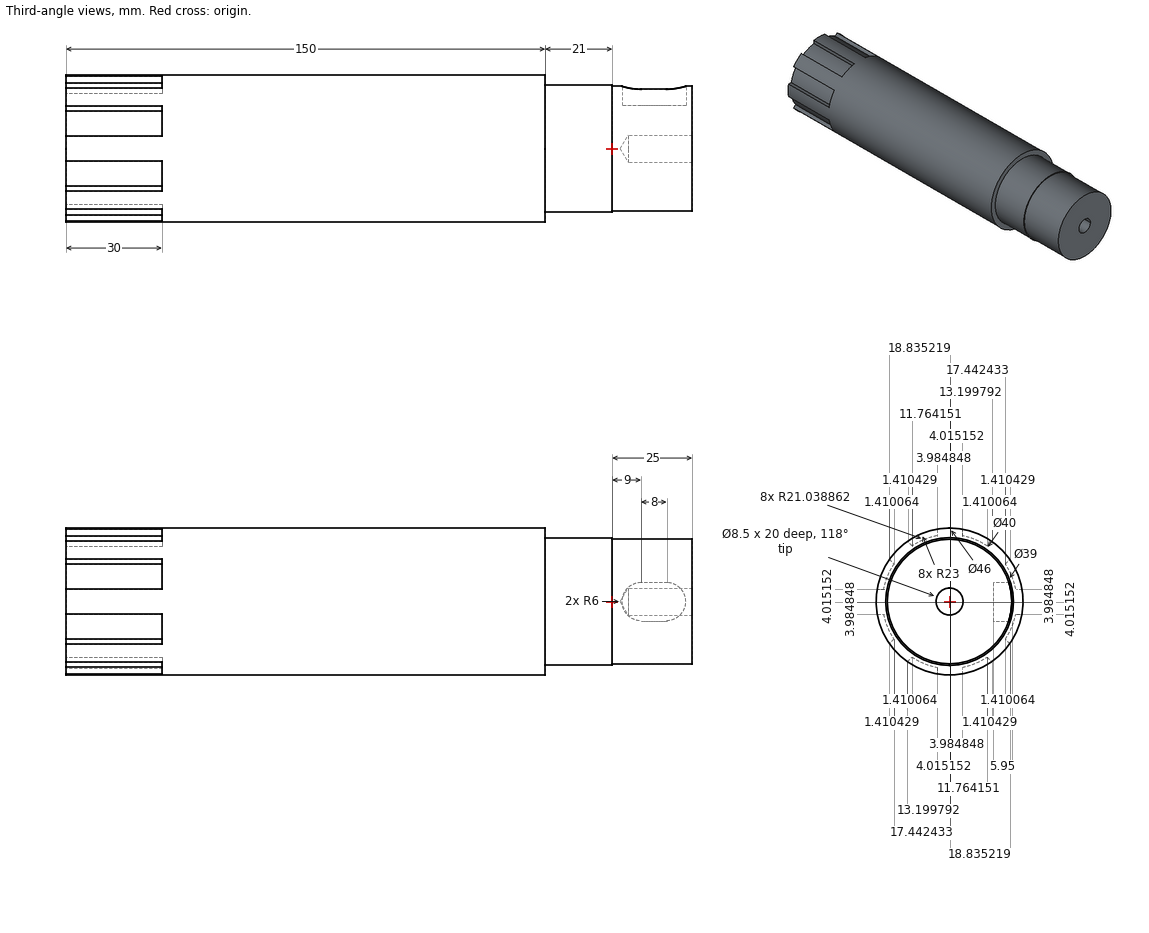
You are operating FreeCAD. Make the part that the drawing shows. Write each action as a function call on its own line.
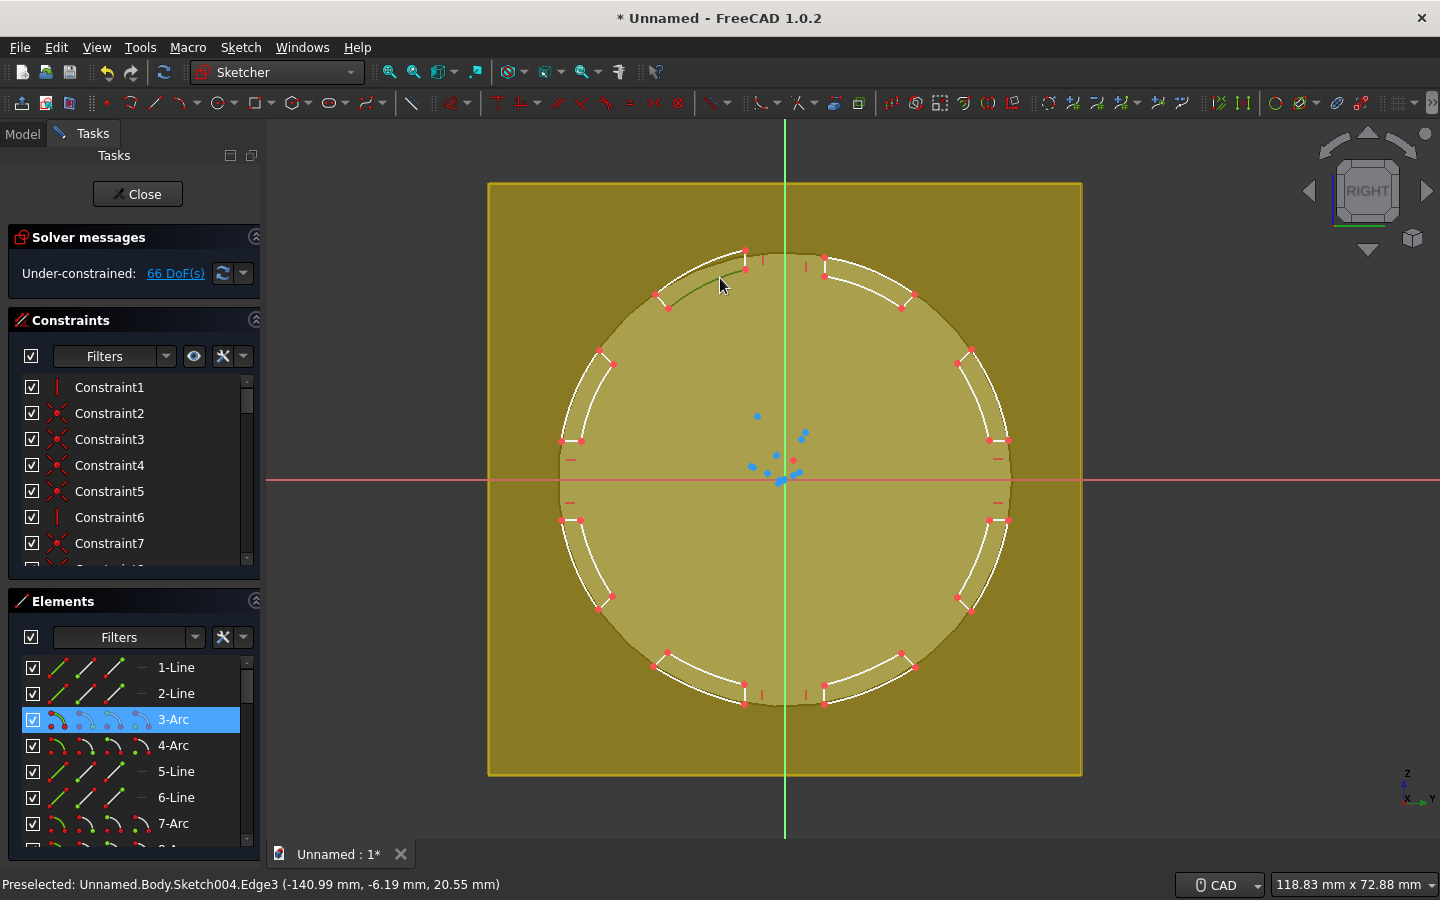
click(680, 681)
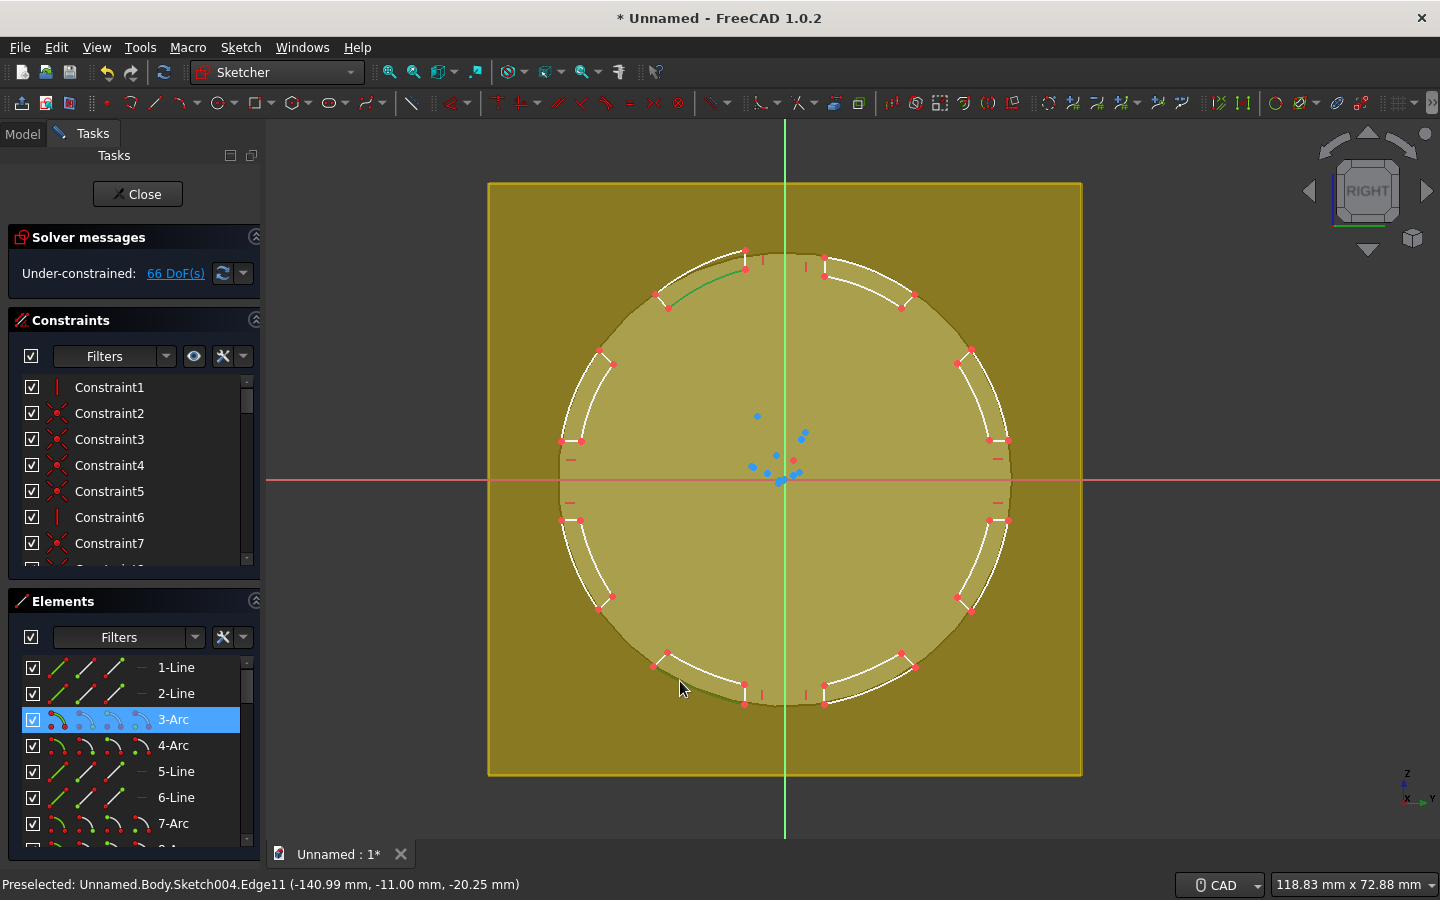
click(498, 104)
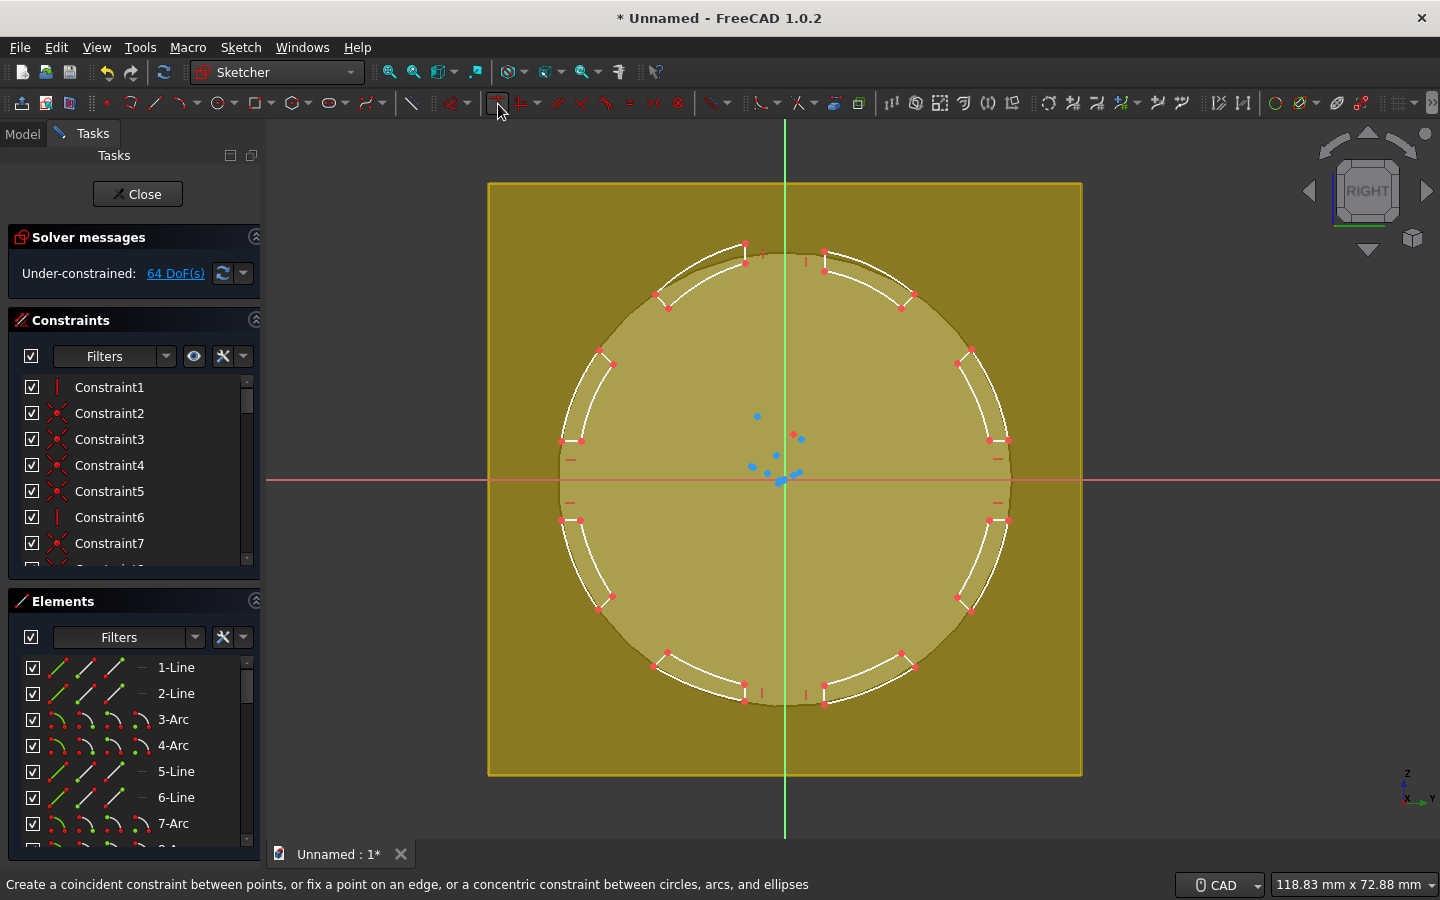
click(720, 273)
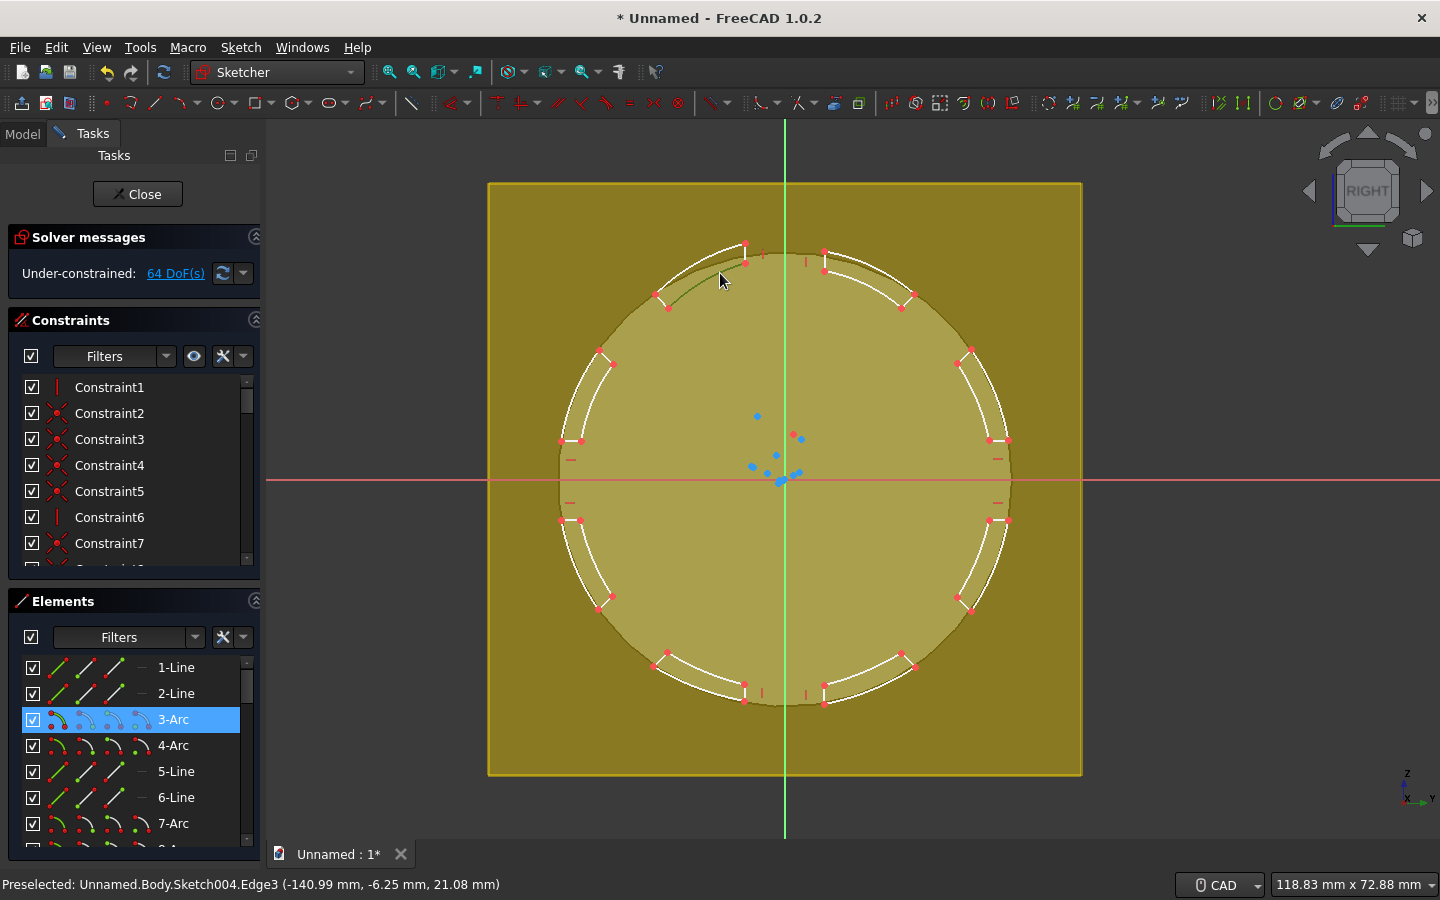
click(690, 665)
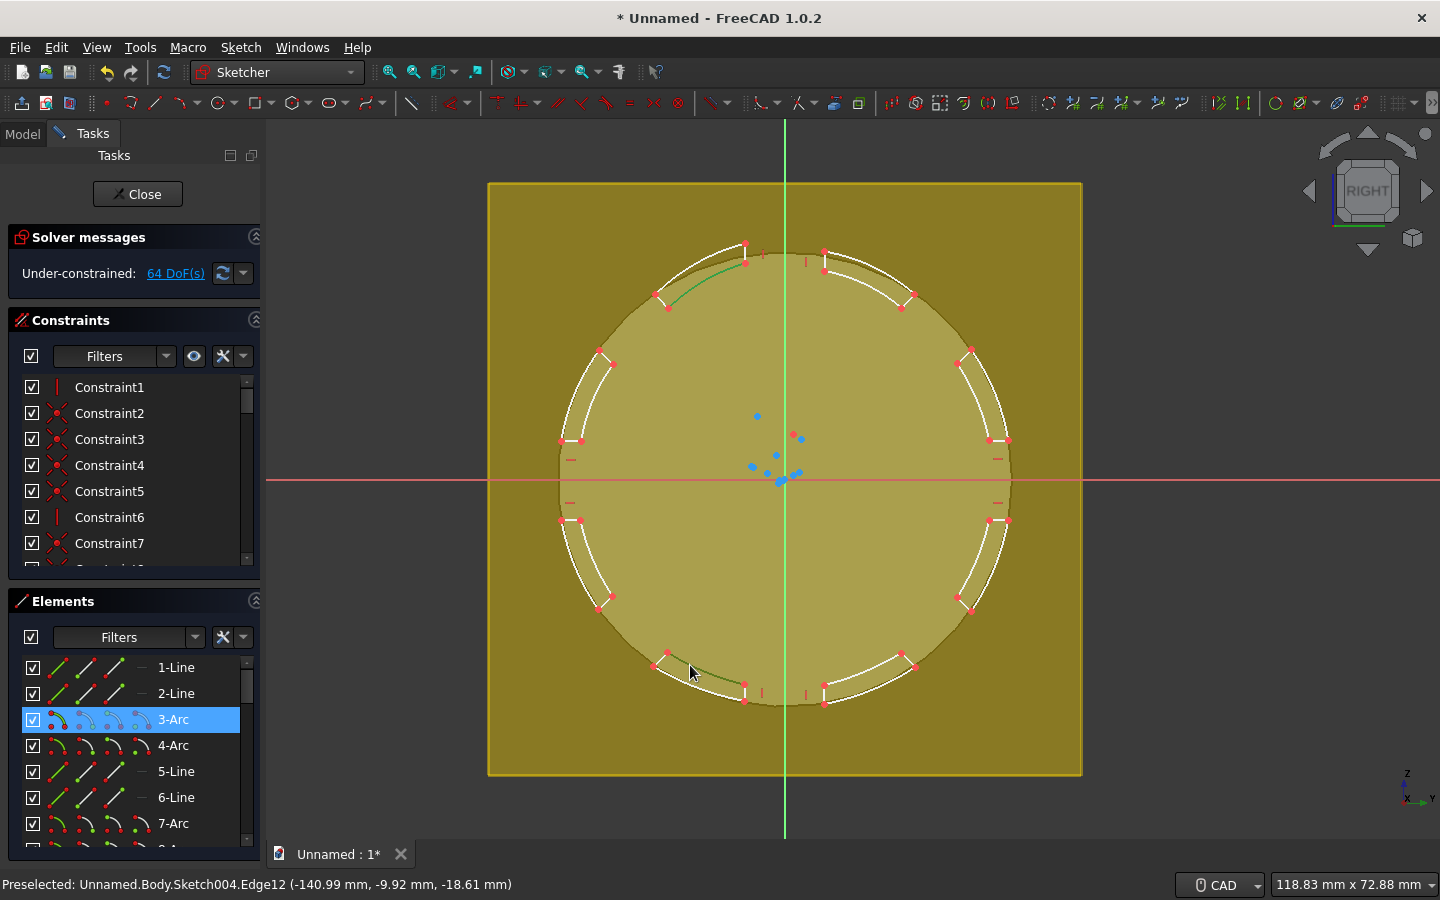
click(498, 104)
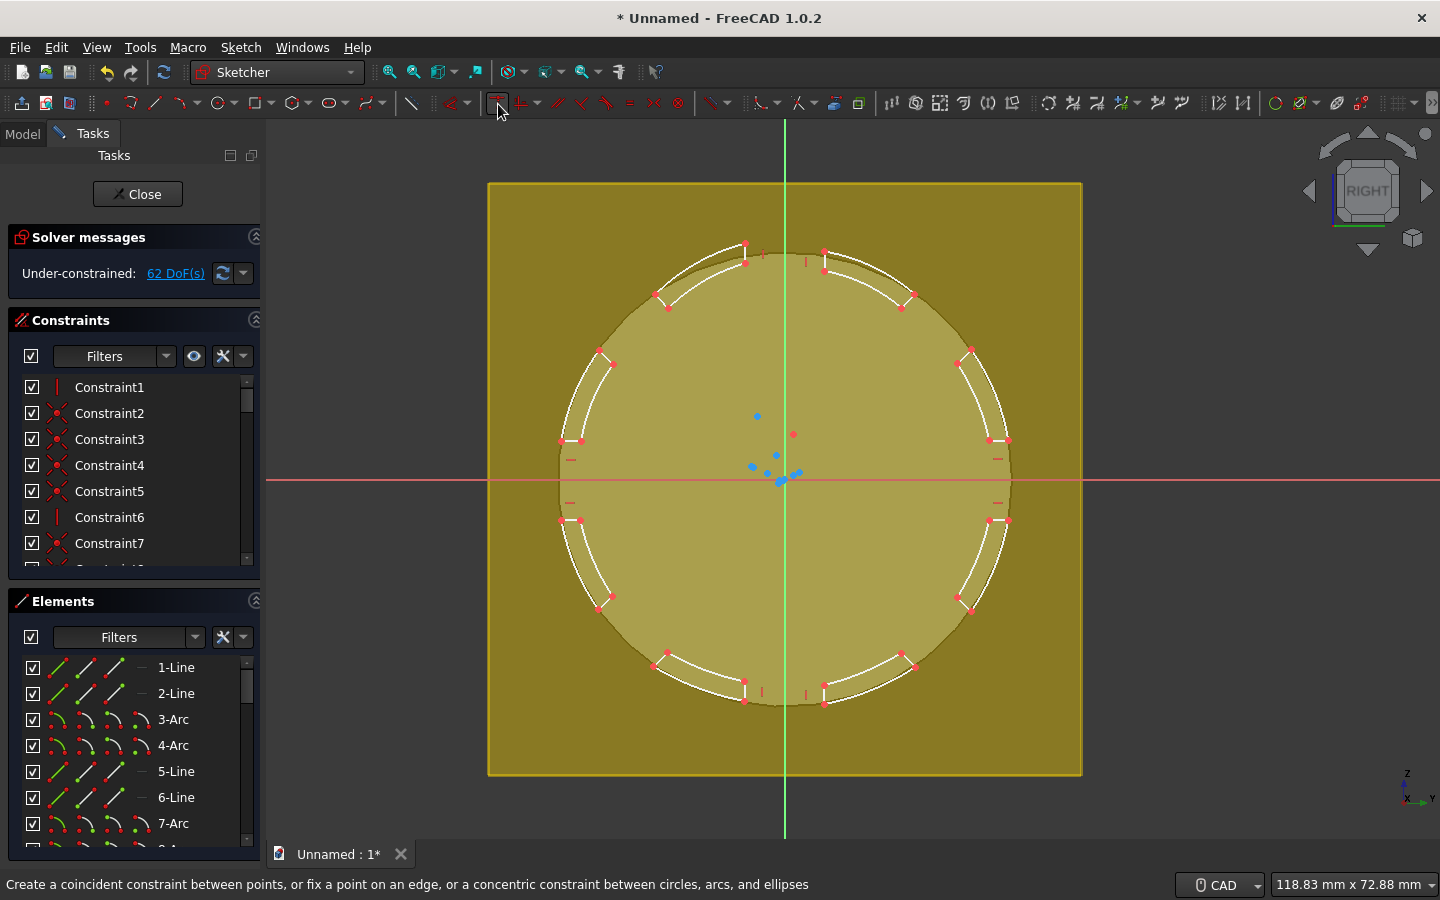
click(720, 273)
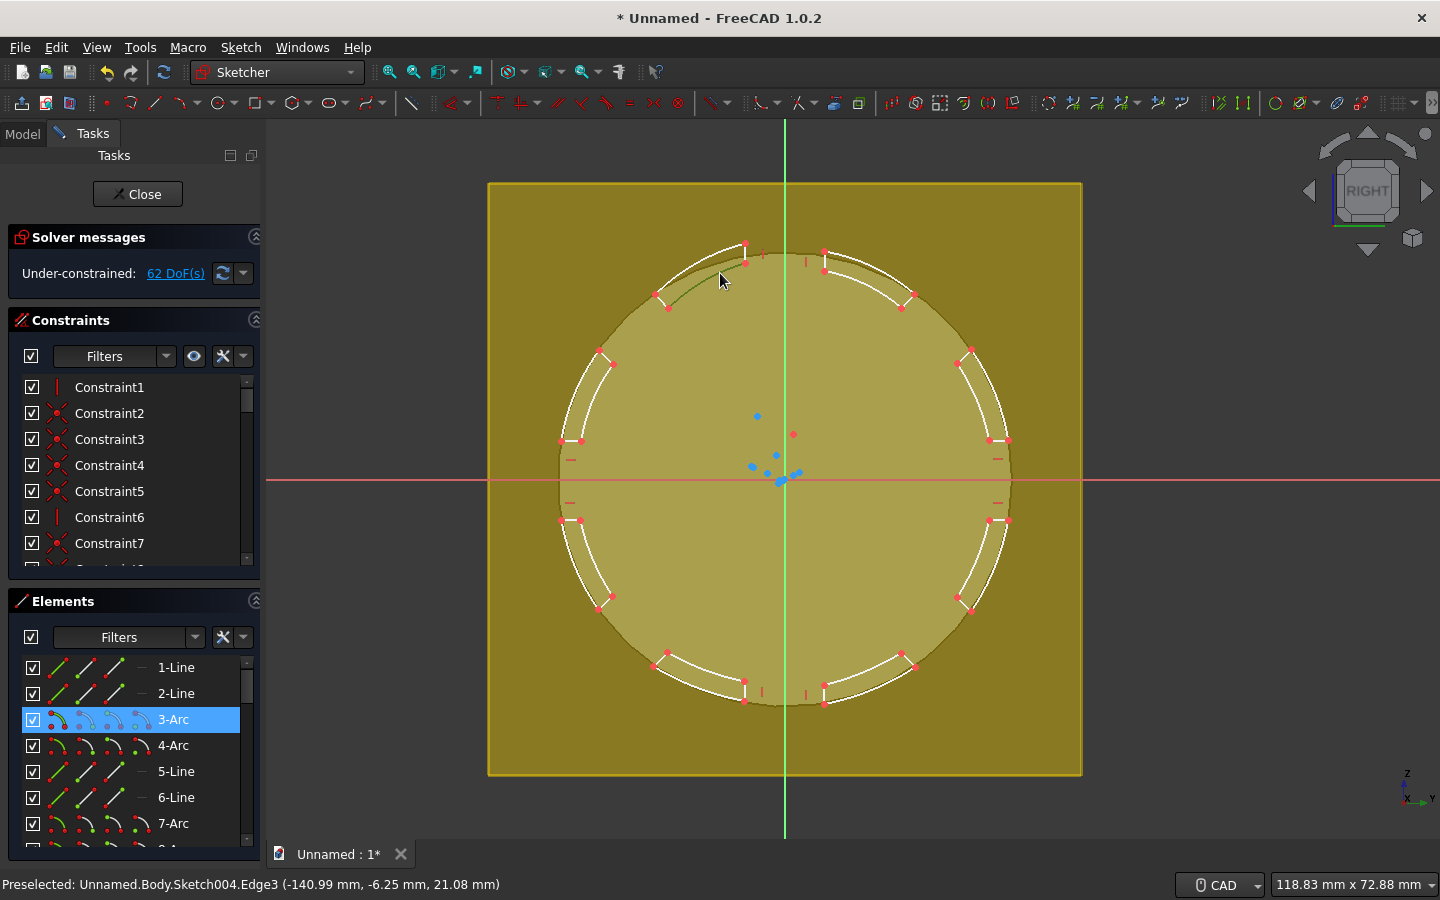
click(568, 549)